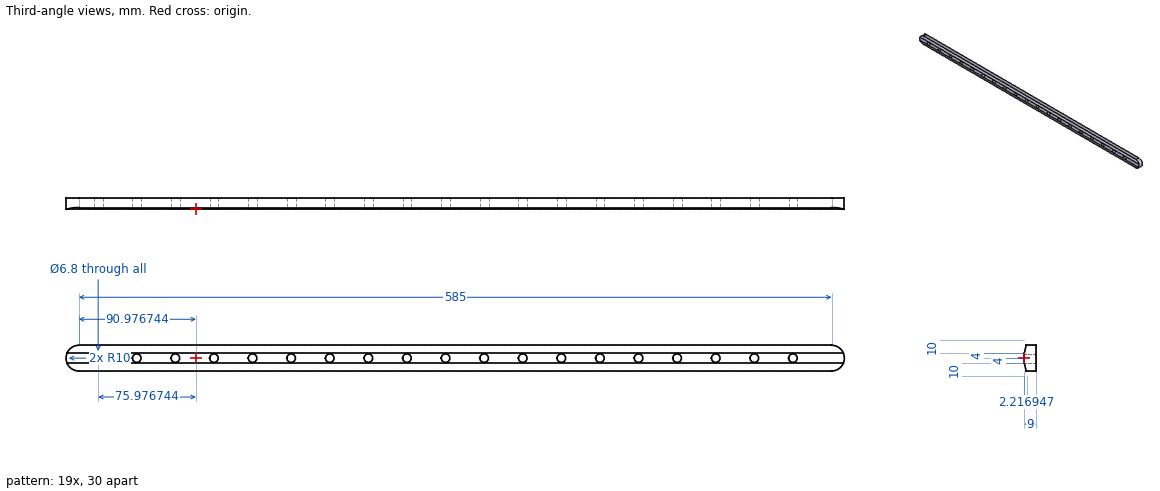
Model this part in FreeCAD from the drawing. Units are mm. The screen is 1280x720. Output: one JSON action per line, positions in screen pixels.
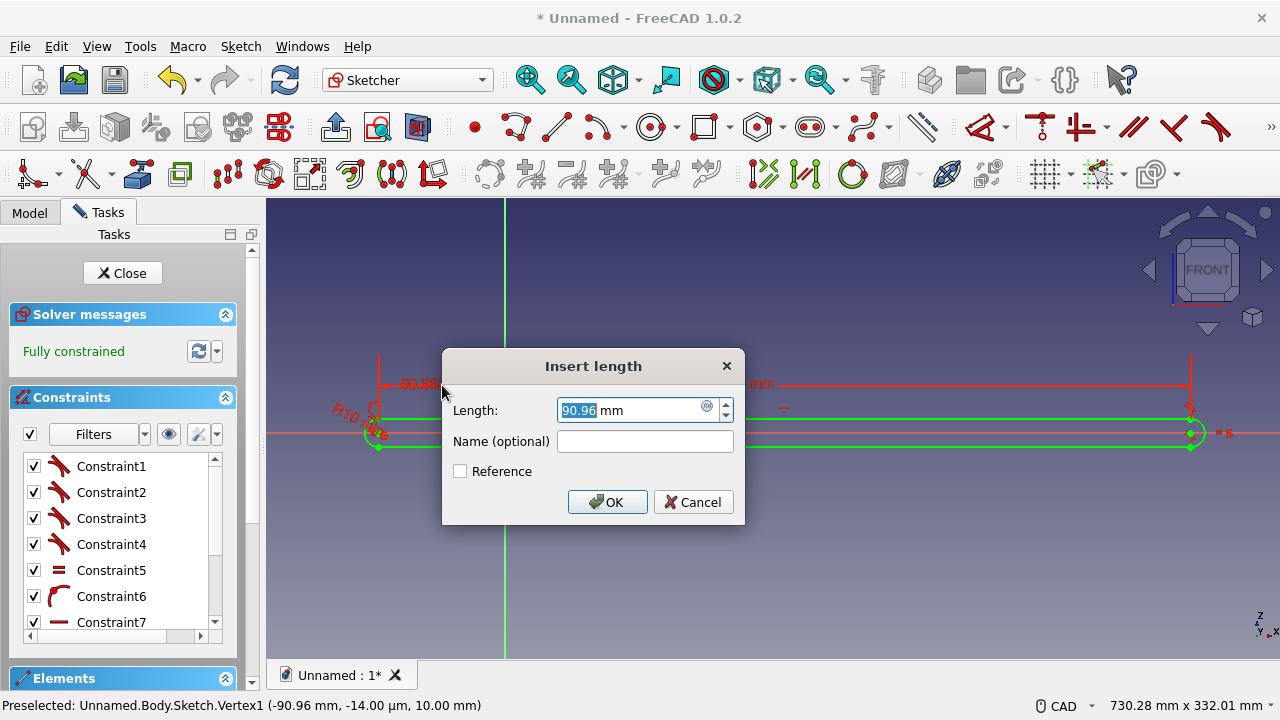
{"action": "type", "text": "90.976744"}
{"action": "key", "text": "Return"}
{"action": "key", "text": "Escape"}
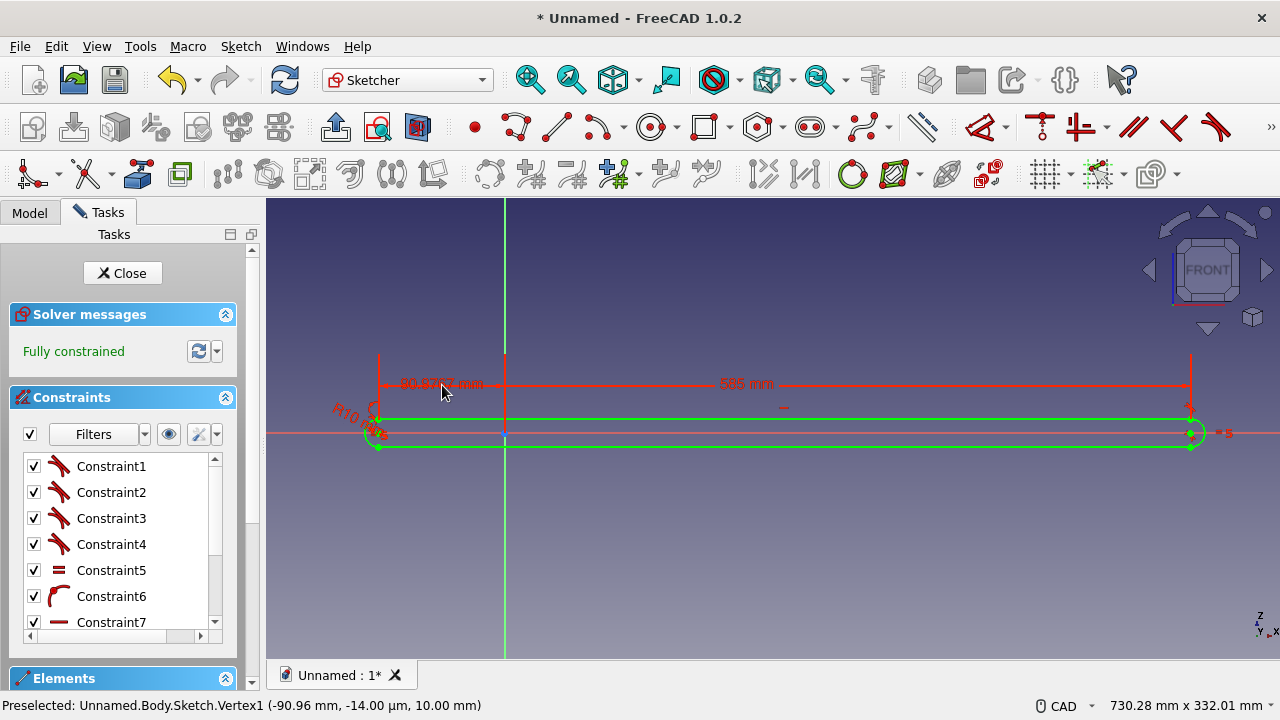
{"action": "left_click", "coordinate": [123, 273]}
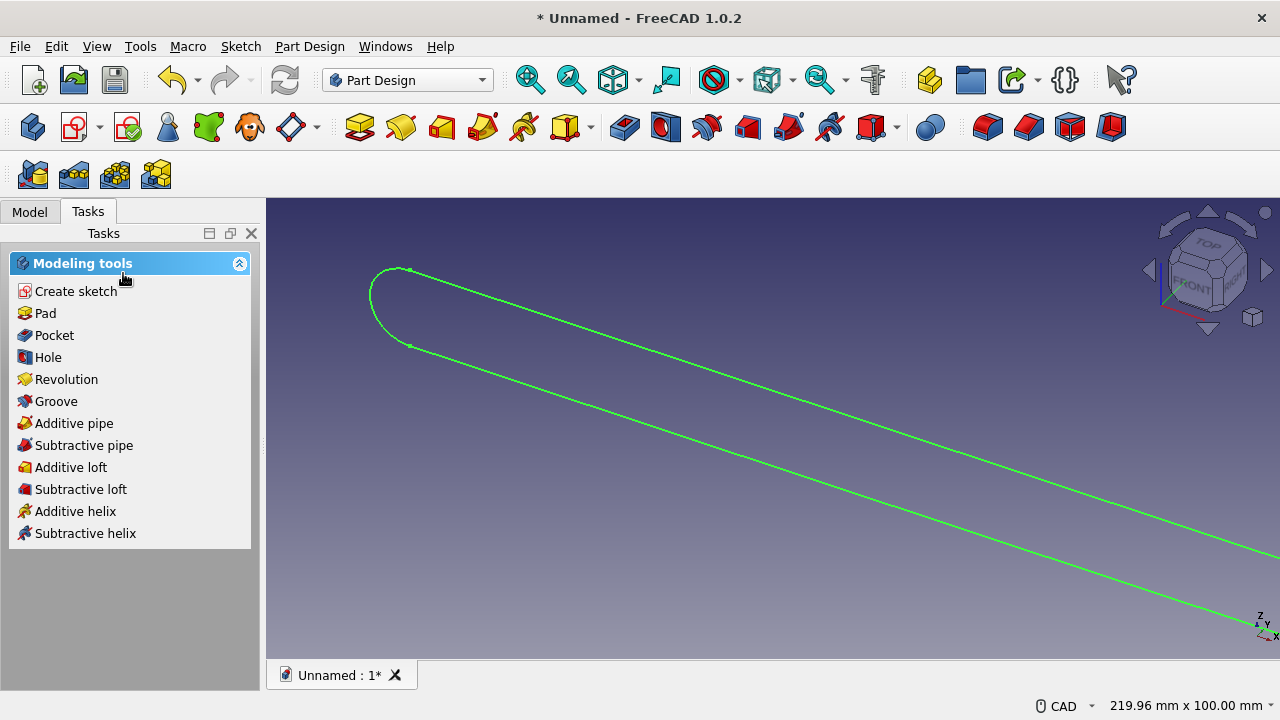
{"action": "left_click", "coordinate": [360, 128]}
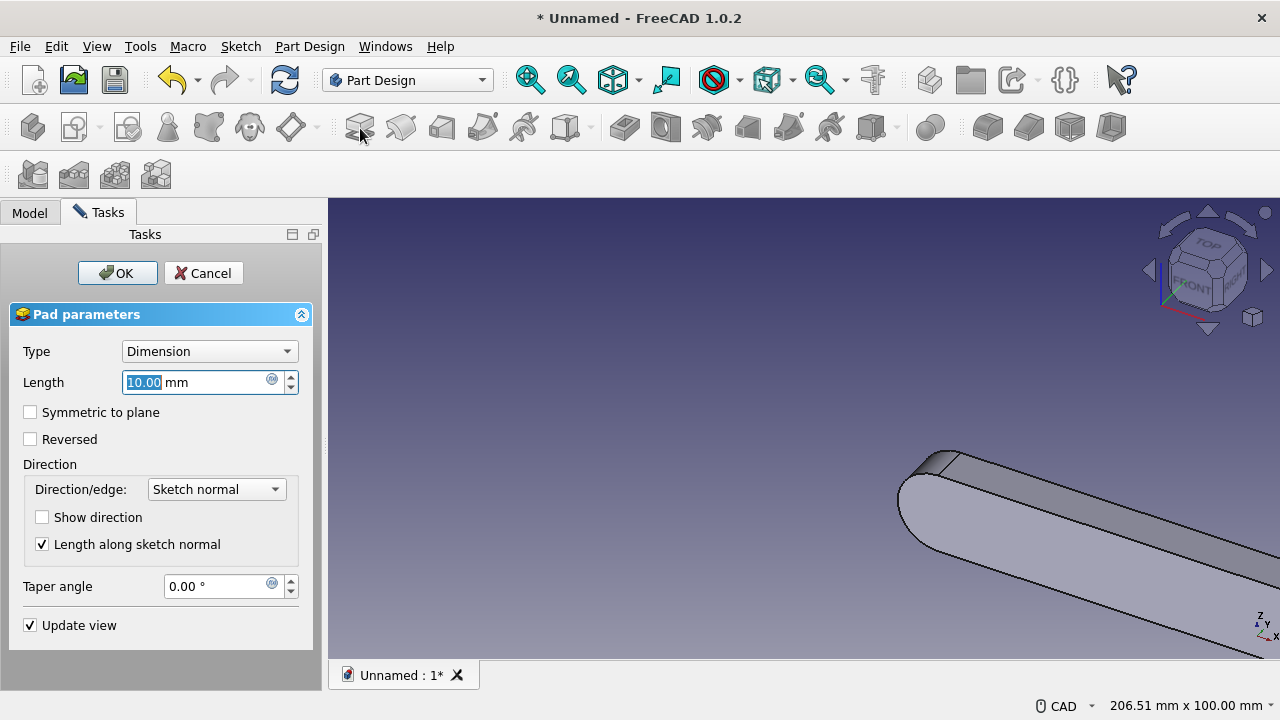
{"action": "type", "text": "9"}
{"action": "key", "text": "Tab"}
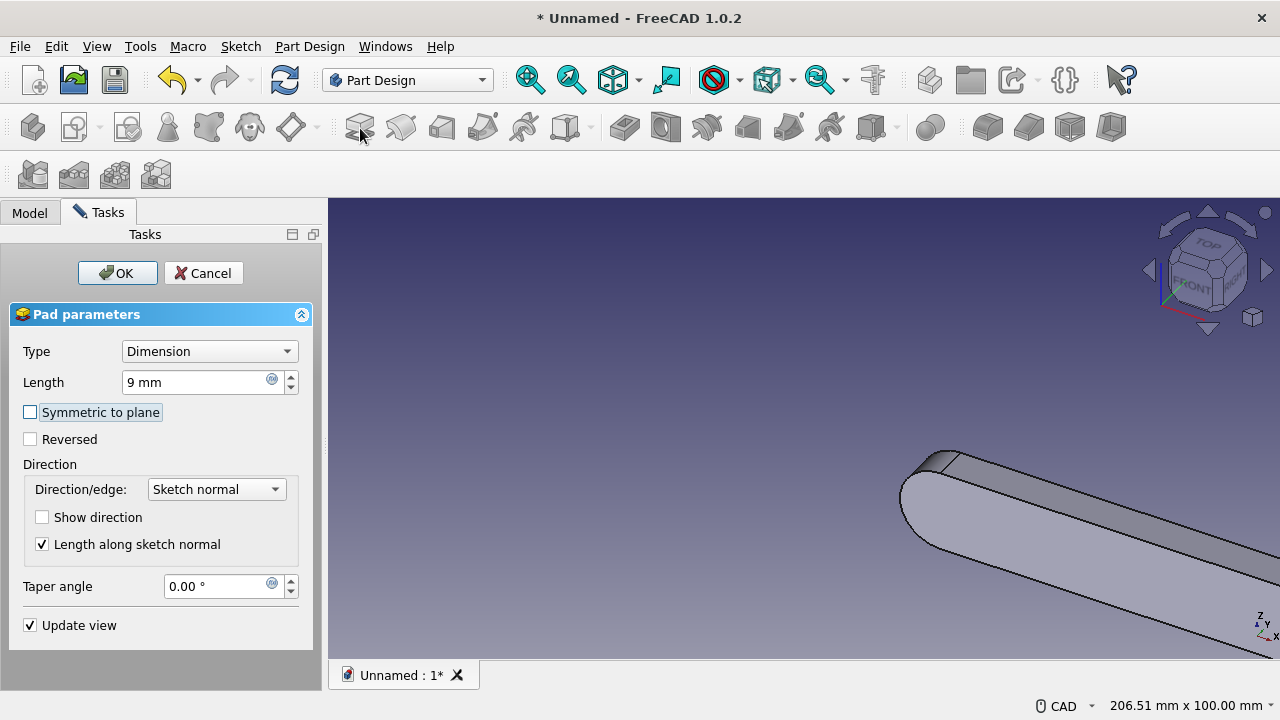
{"action": "left_click", "coordinate": [31, 439]}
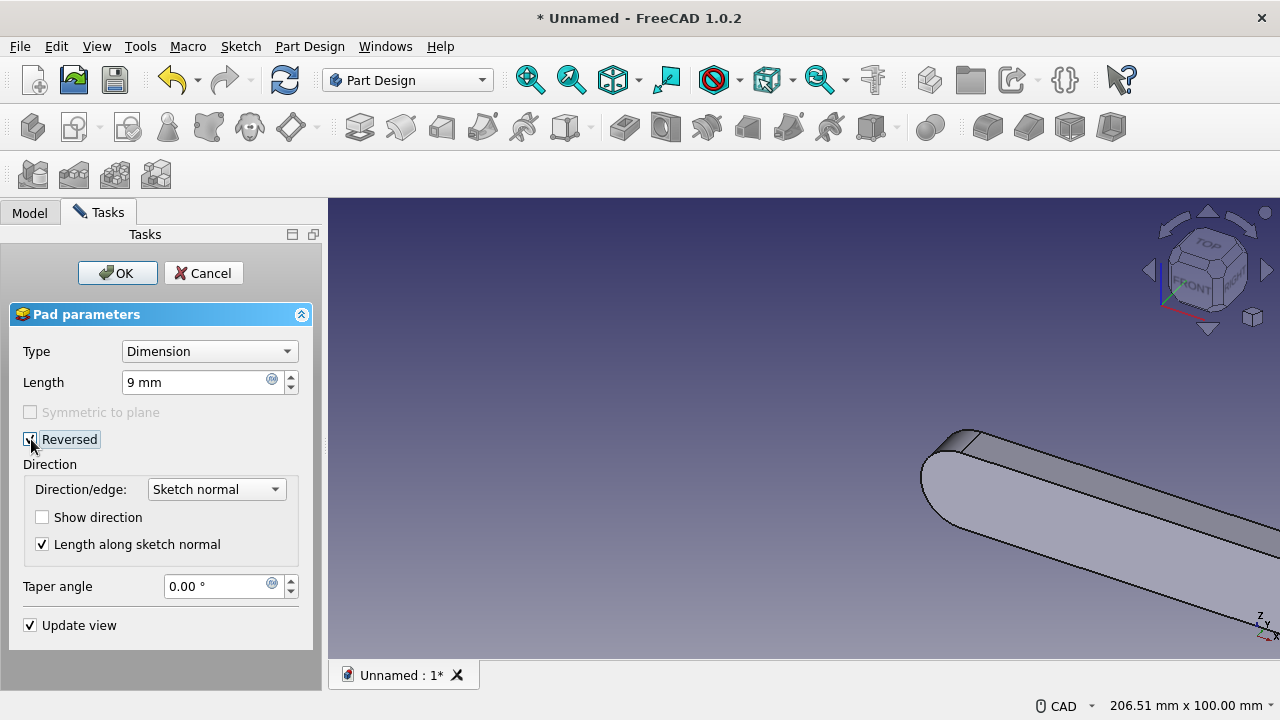
{"action": "left_click", "coordinate": [118, 273]}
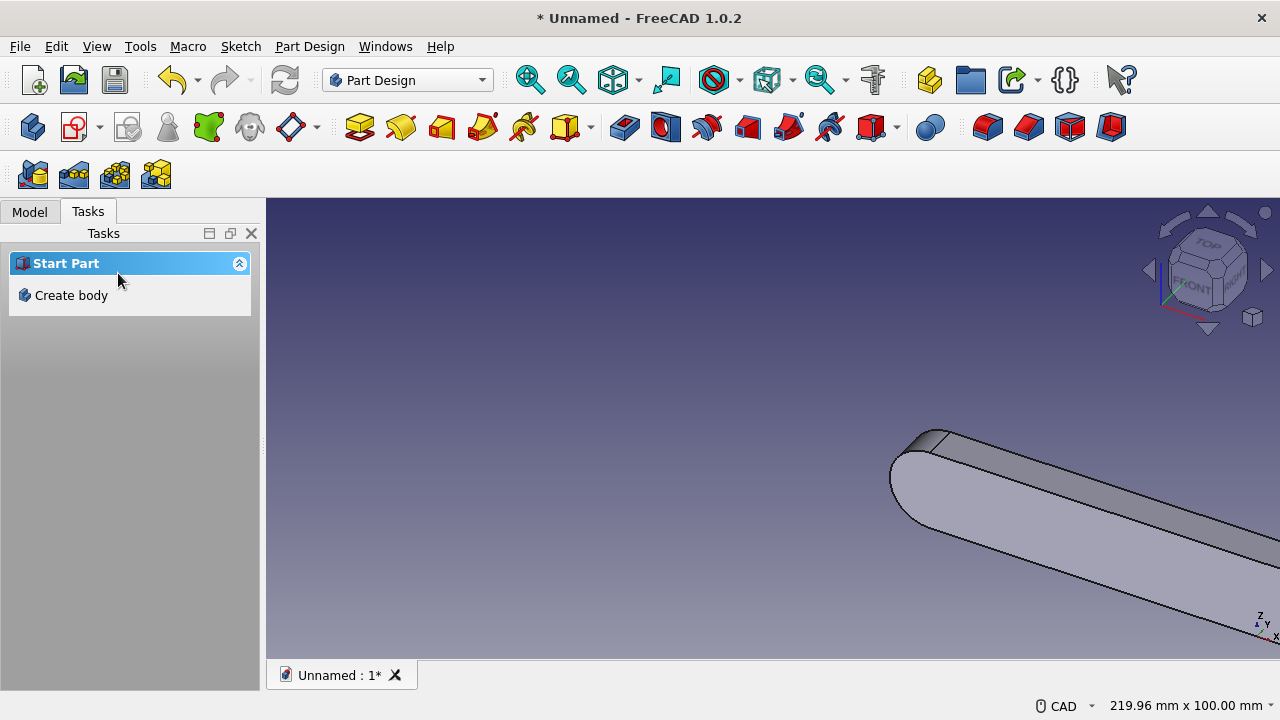
{"action": "left_click", "coordinate": [531, 80]}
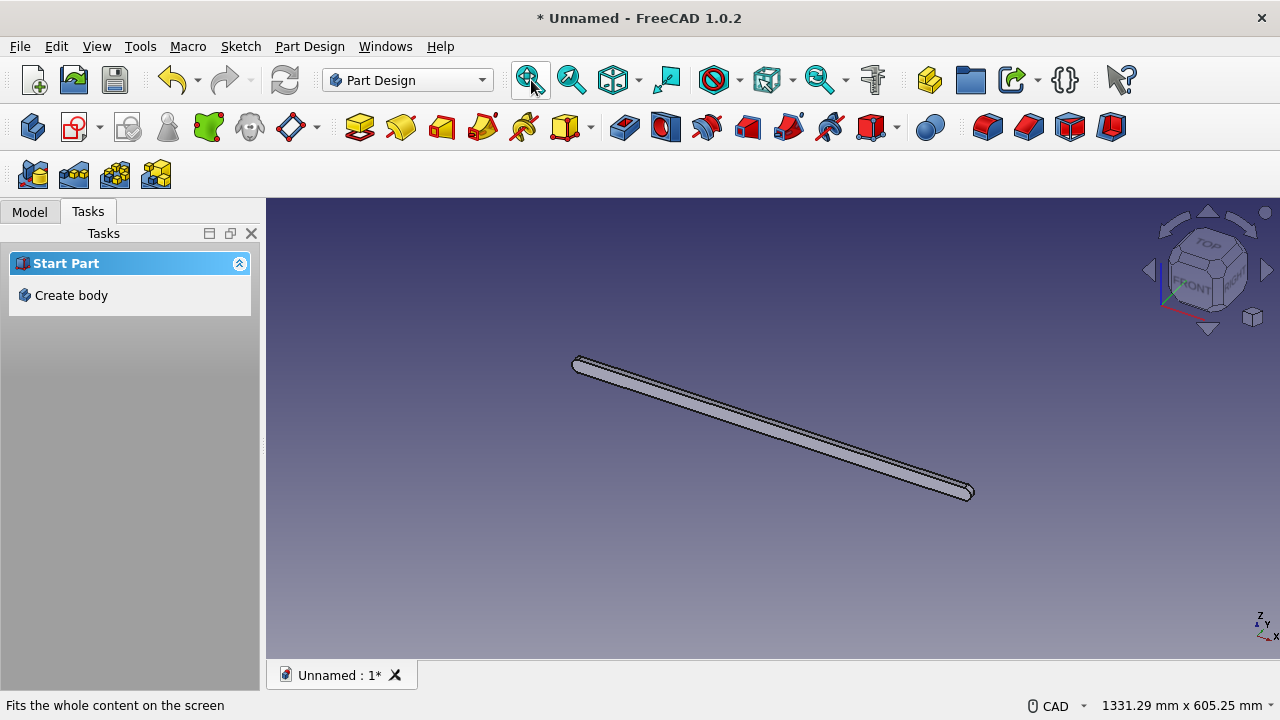
{"action": "key", "text": "4"}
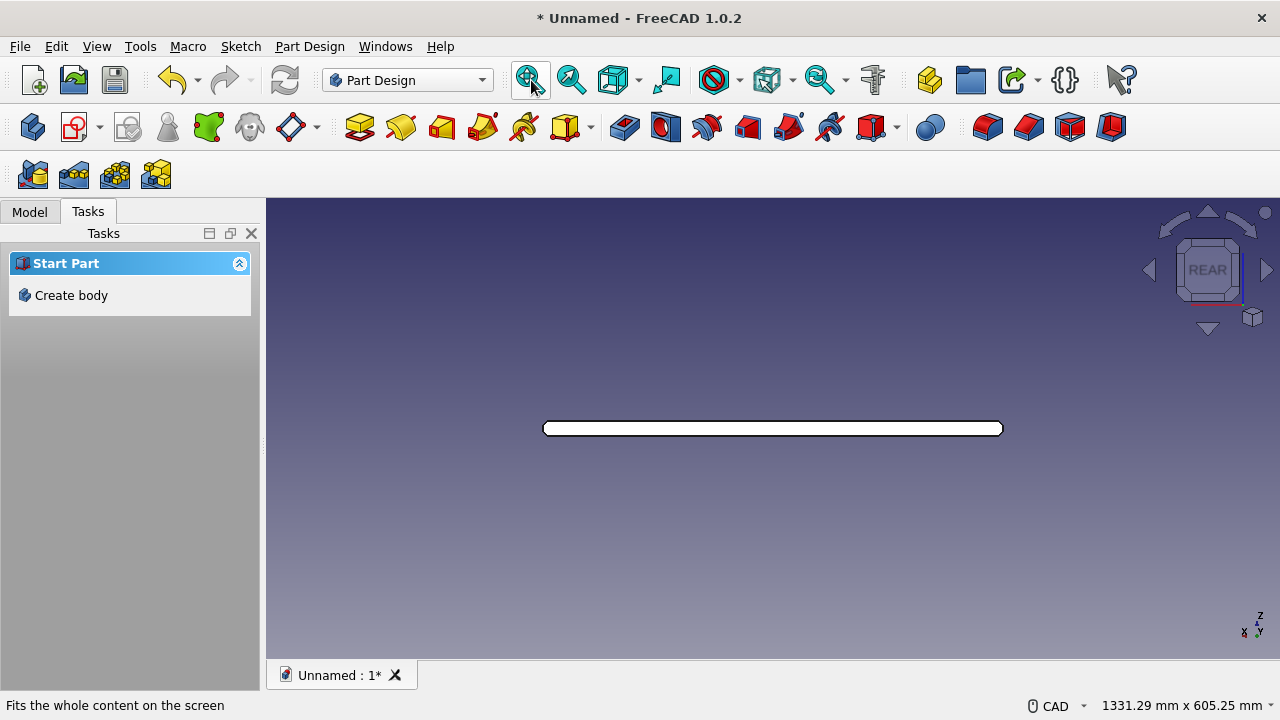
{"action": "left_click", "coordinate": [576, 427]}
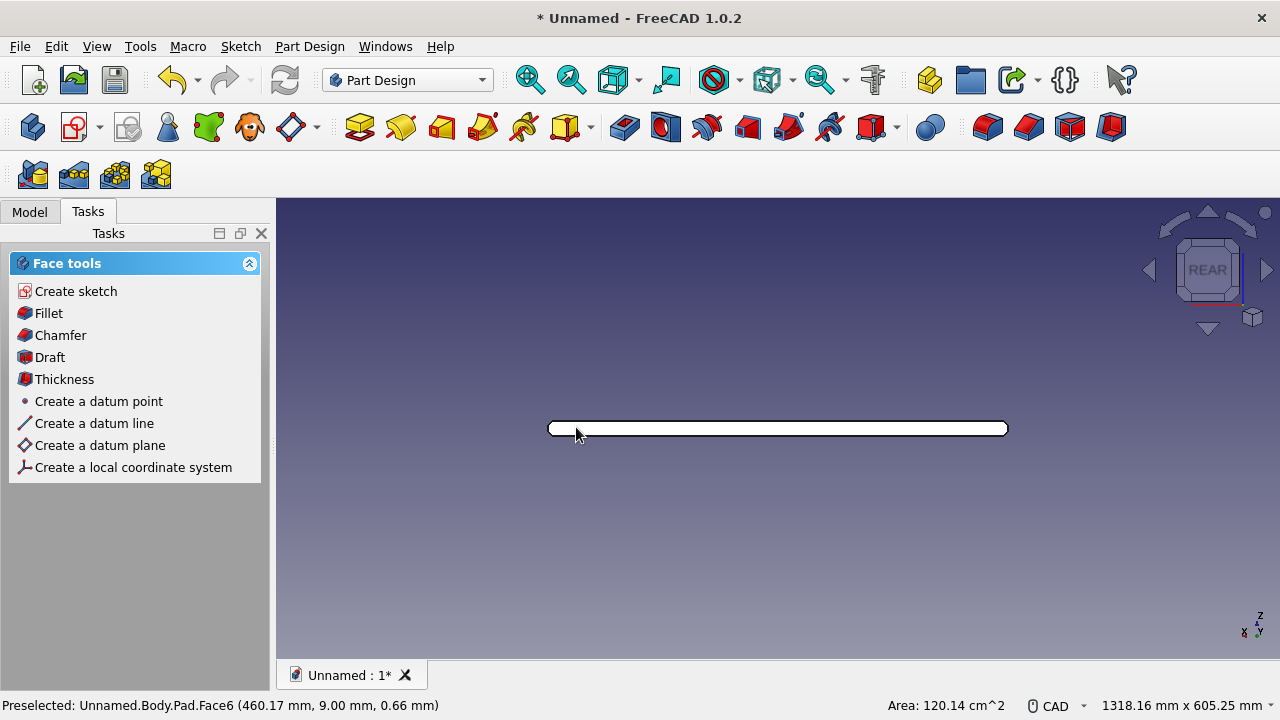
{"action": "left_click", "coordinate": [74, 128]}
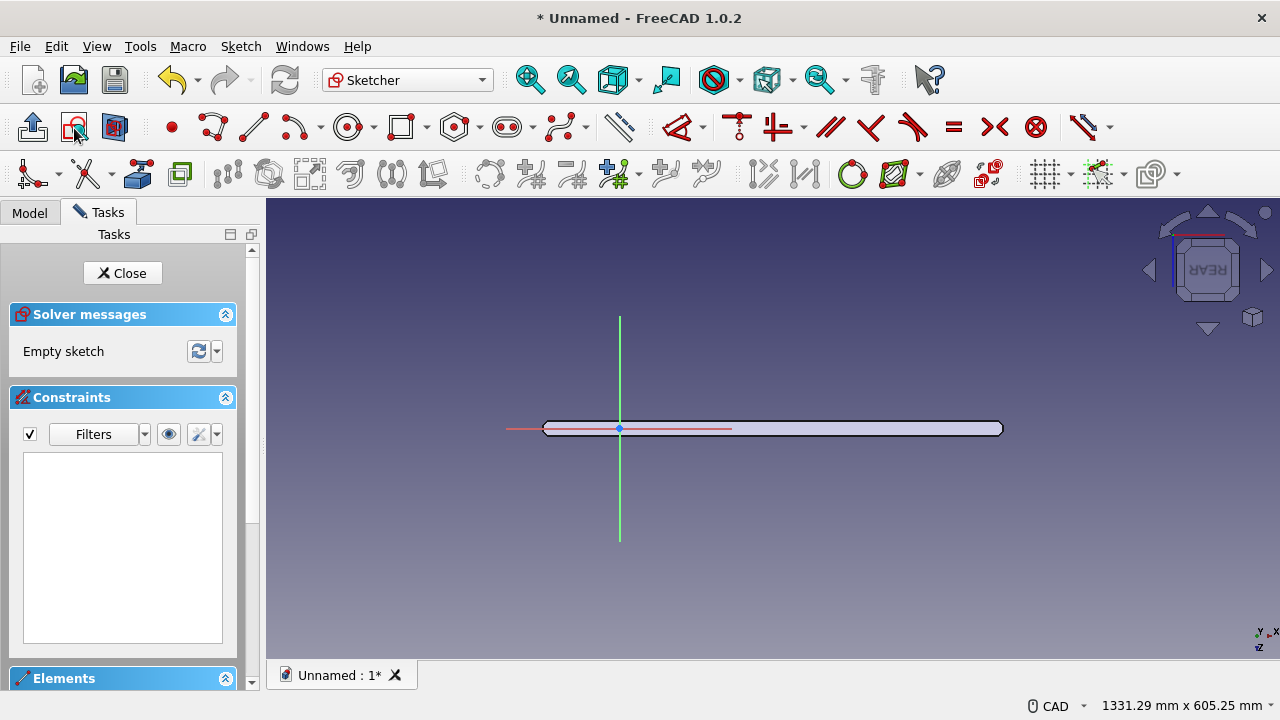
{"action": "scroll", "coordinate": [554, 429], "scroll_direction": "up", "scroll_amount": 15}